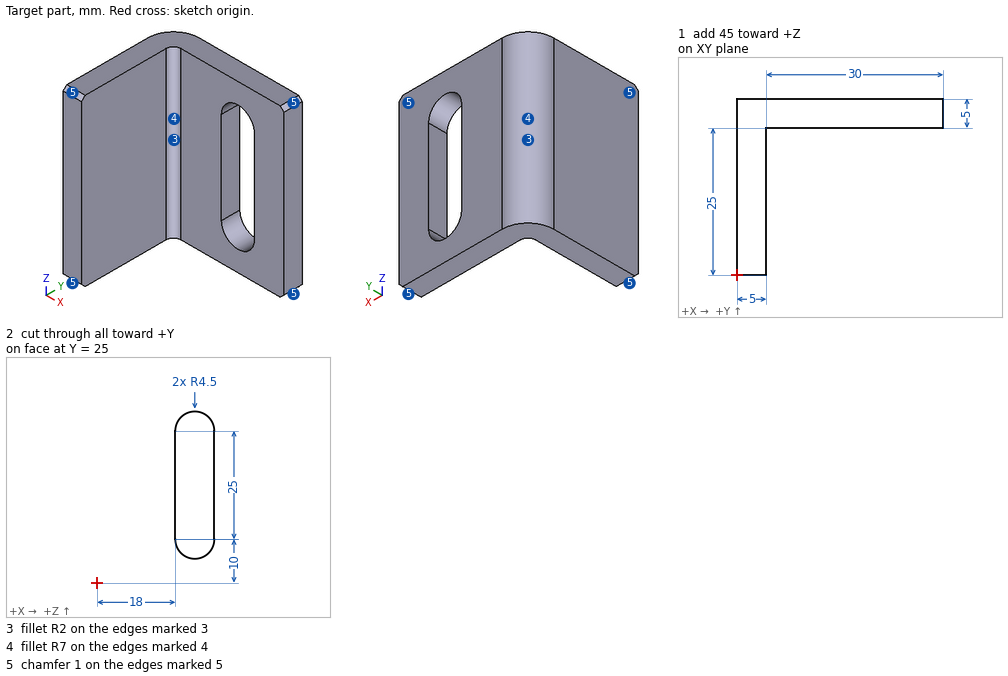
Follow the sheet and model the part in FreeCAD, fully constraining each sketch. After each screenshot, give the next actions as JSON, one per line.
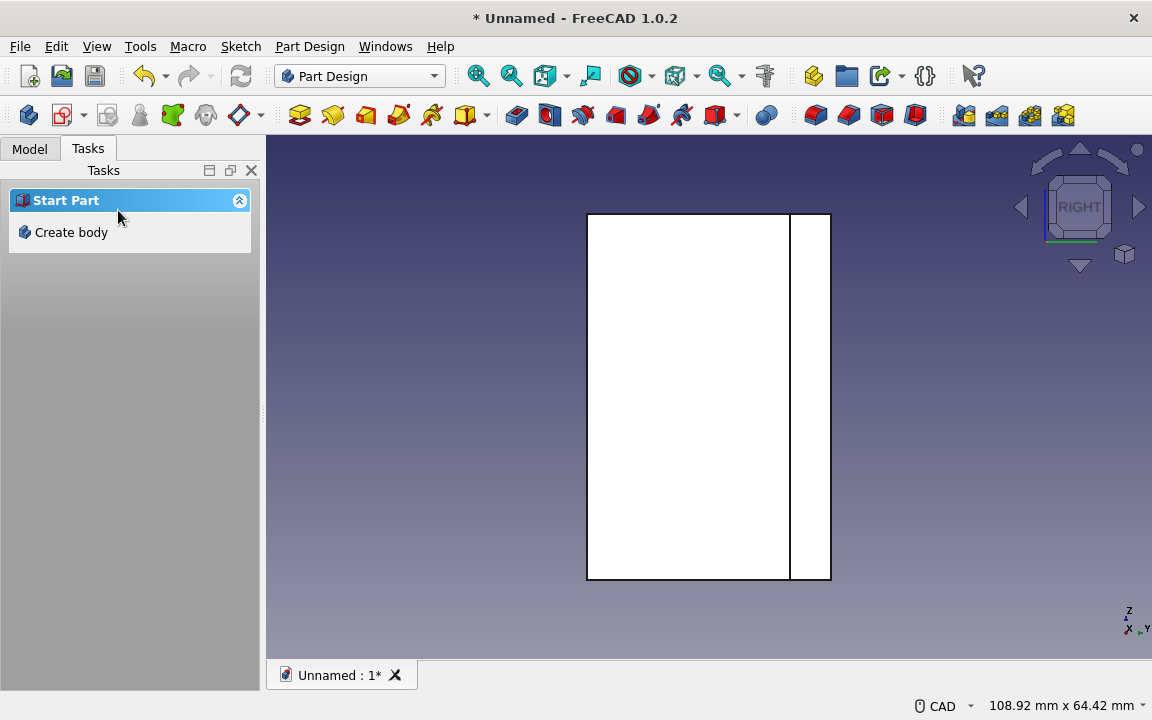
{"action": "key", "text": "5"}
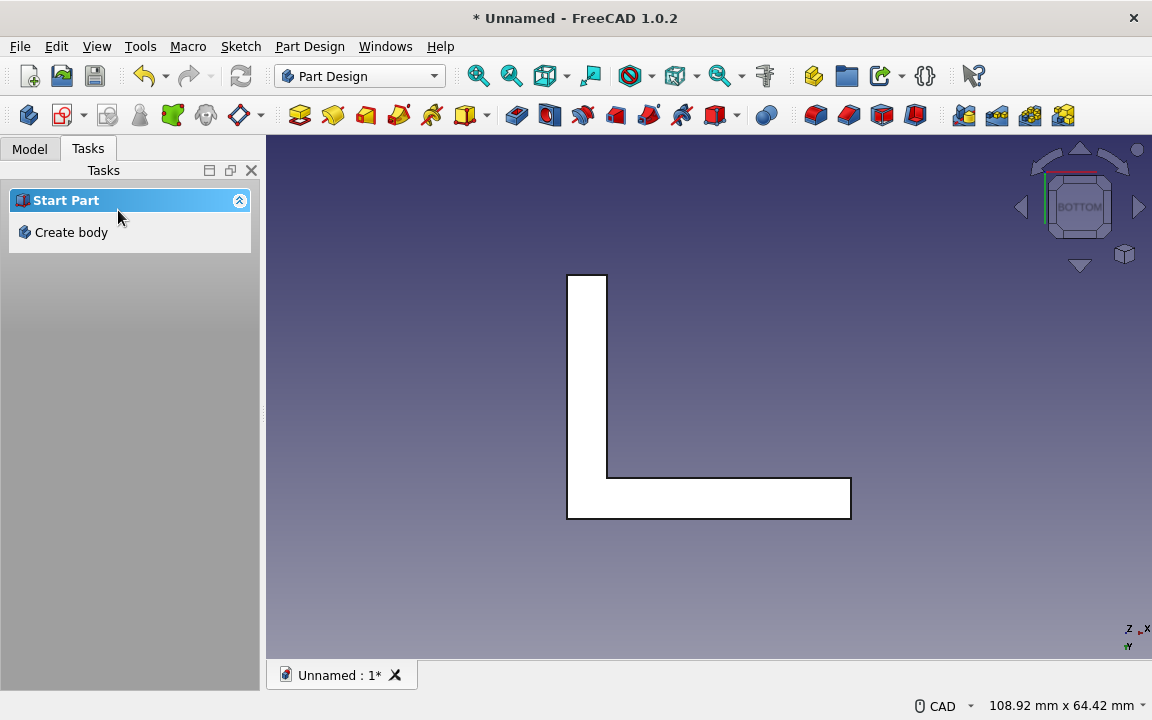
{"action": "key", "text": "4"}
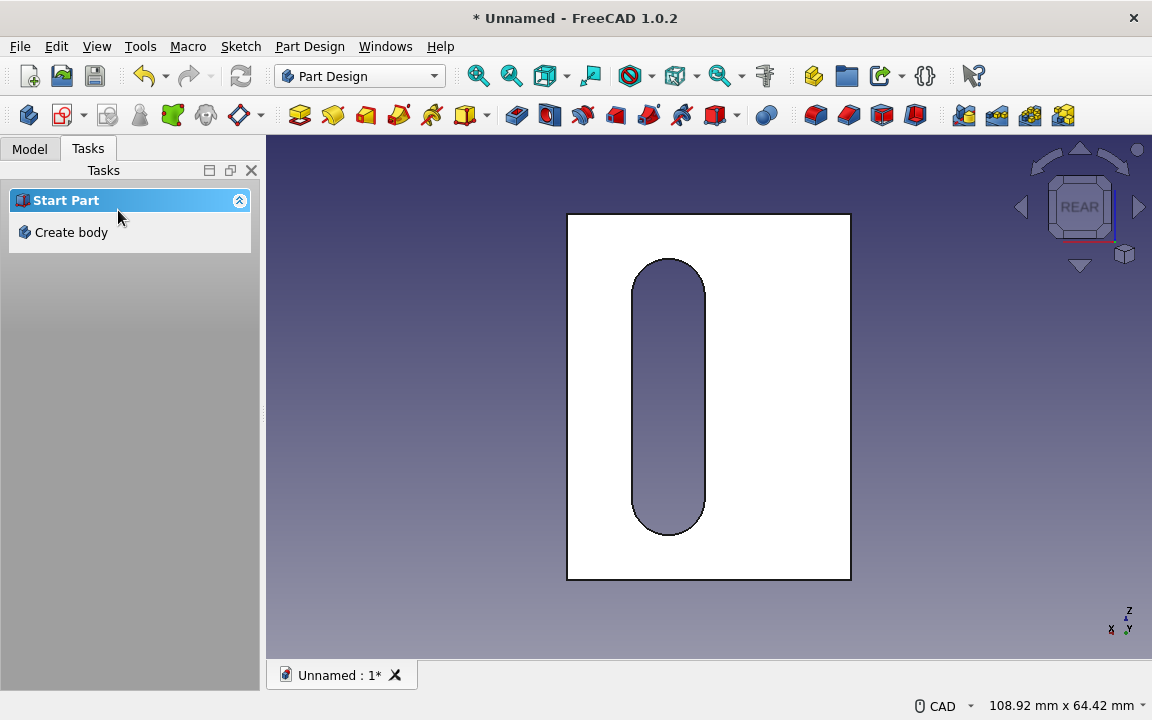
{"action": "key", "text": "6"}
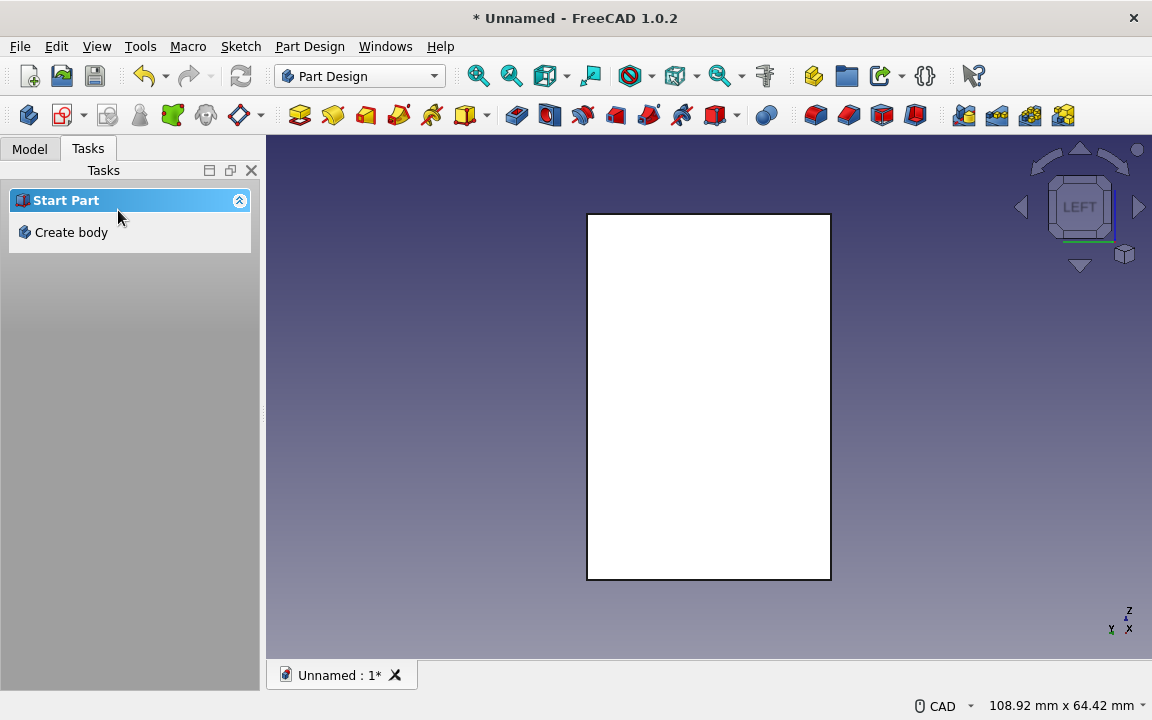
{"action": "key", "text": "v 3"}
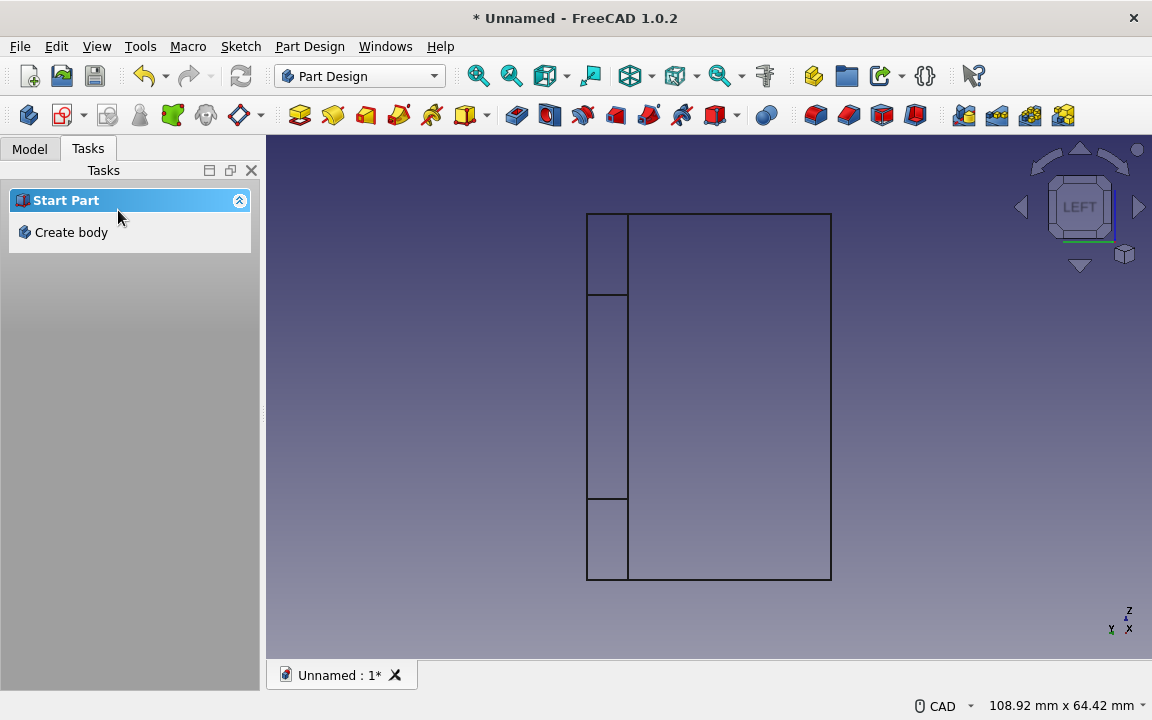
{"action": "key", "text": "0"}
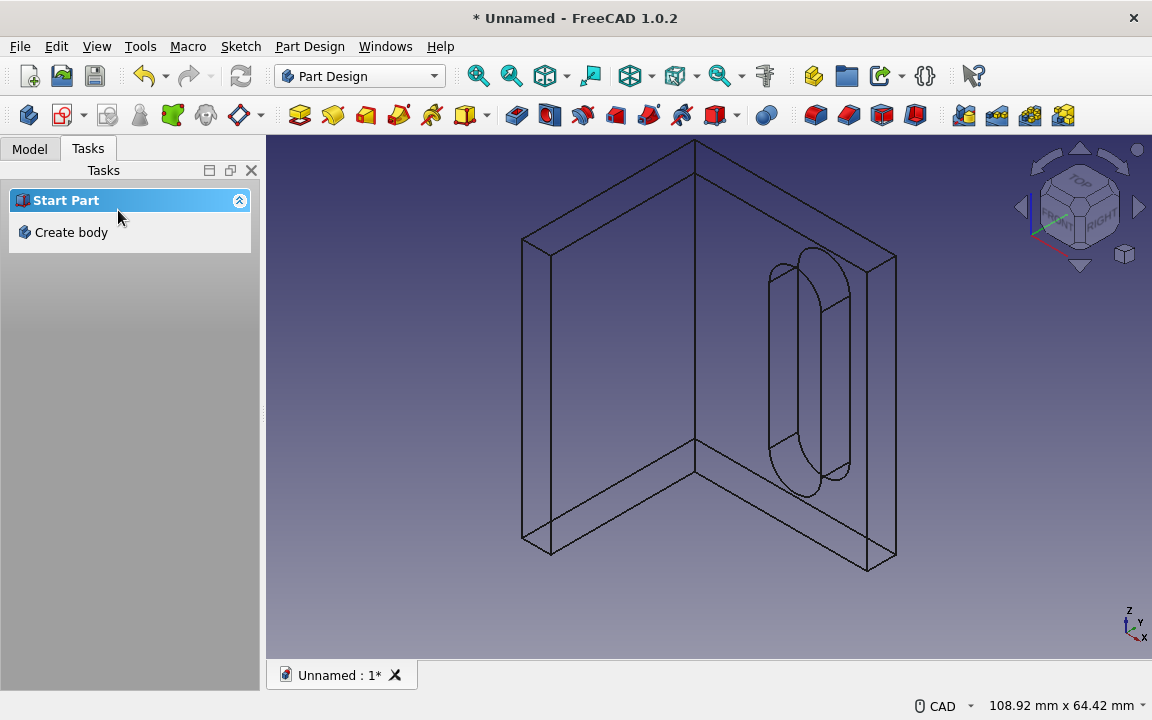
{"action": "left_click", "coordinate": [695, 321]}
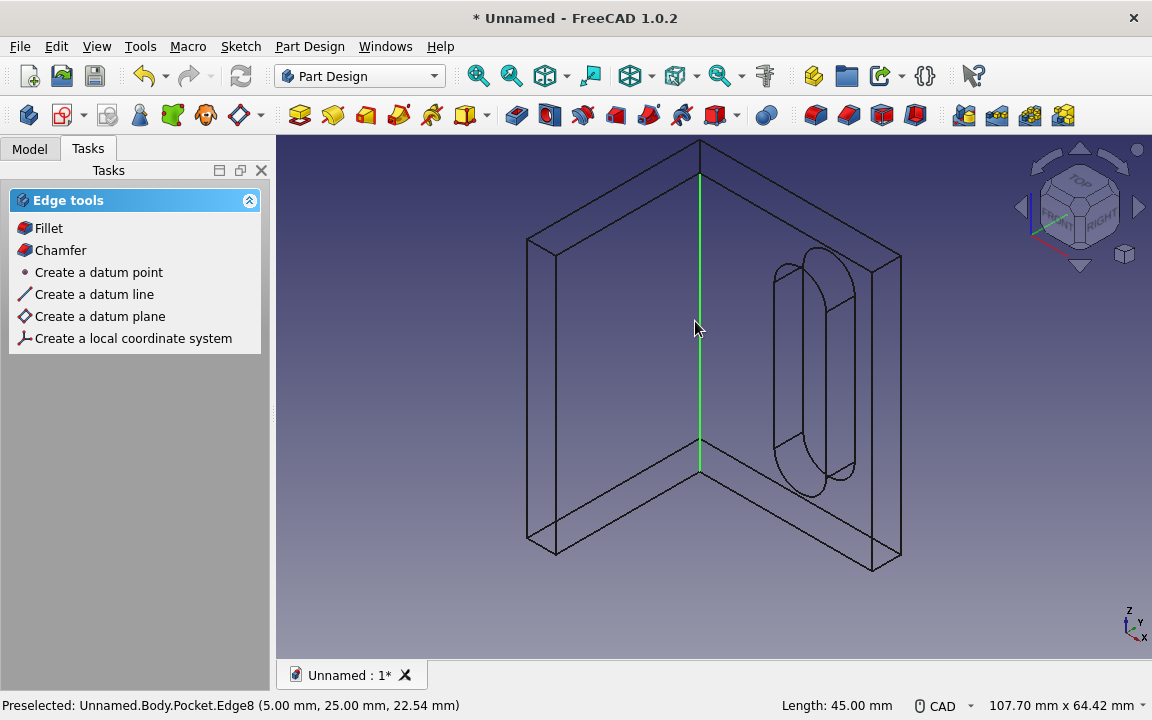
{"action": "key", "text": "v 1"}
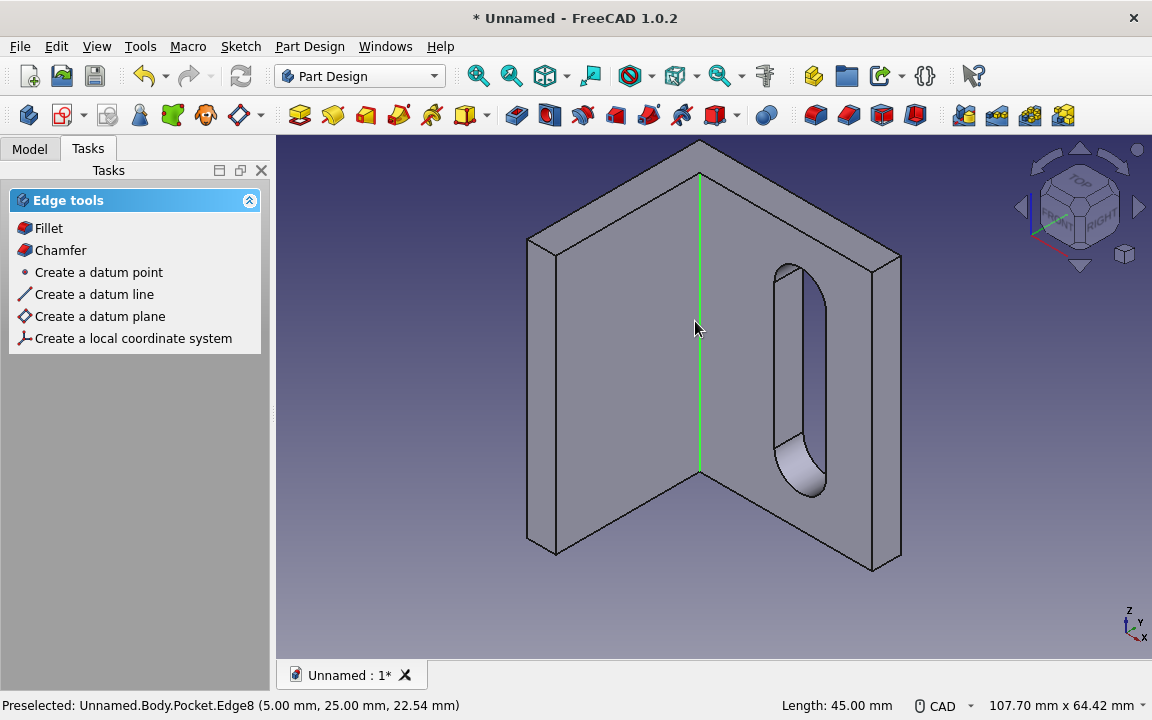
{"action": "left_click", "coordinate": [816, 116]}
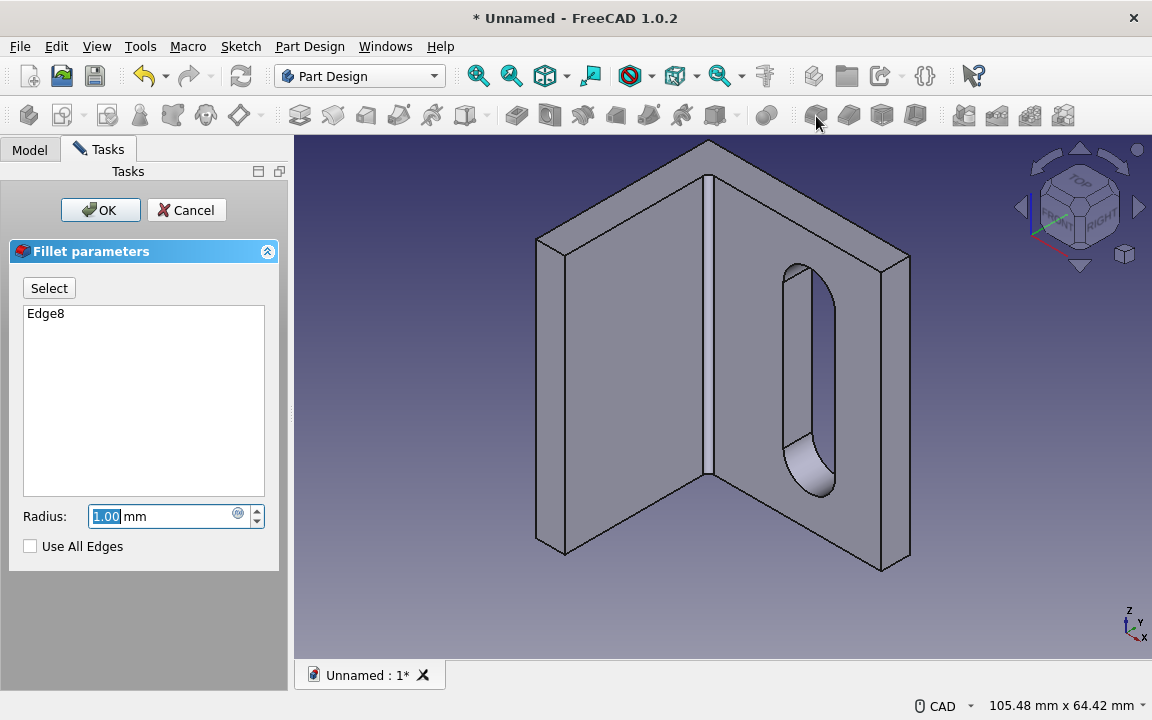
{"action": "type", "text": "2"}
{"action": "key", "text": "Tab"}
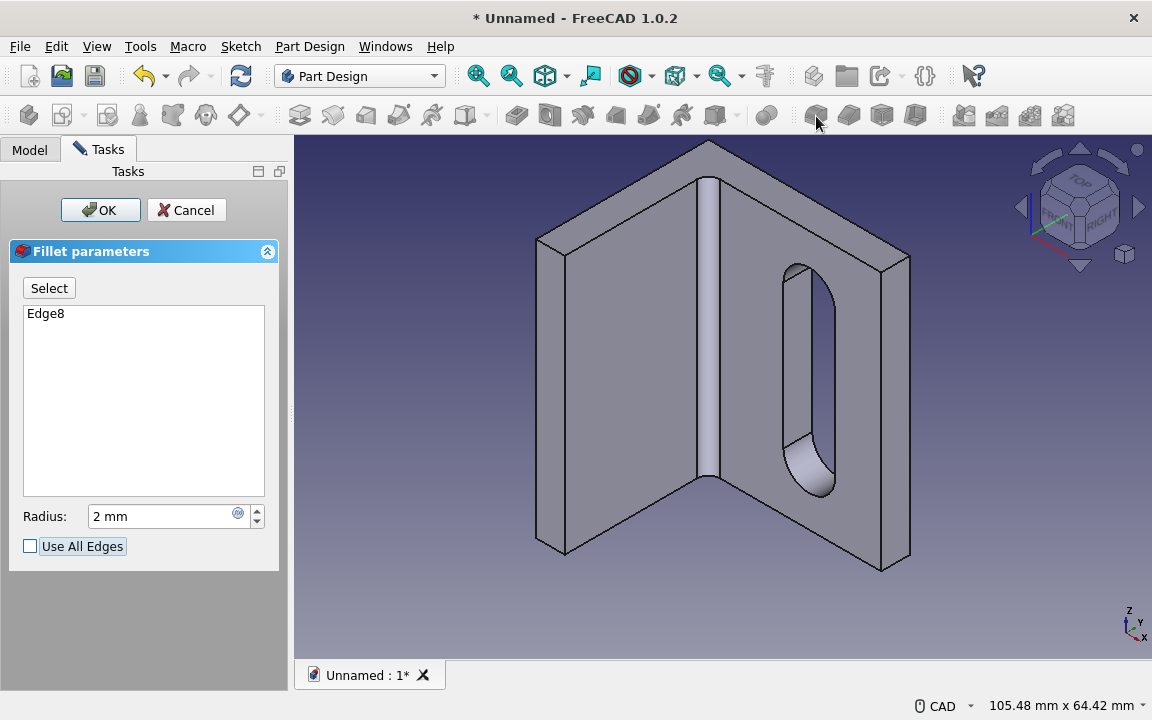
{"action": "left_click", "coordinate": [101, 210]}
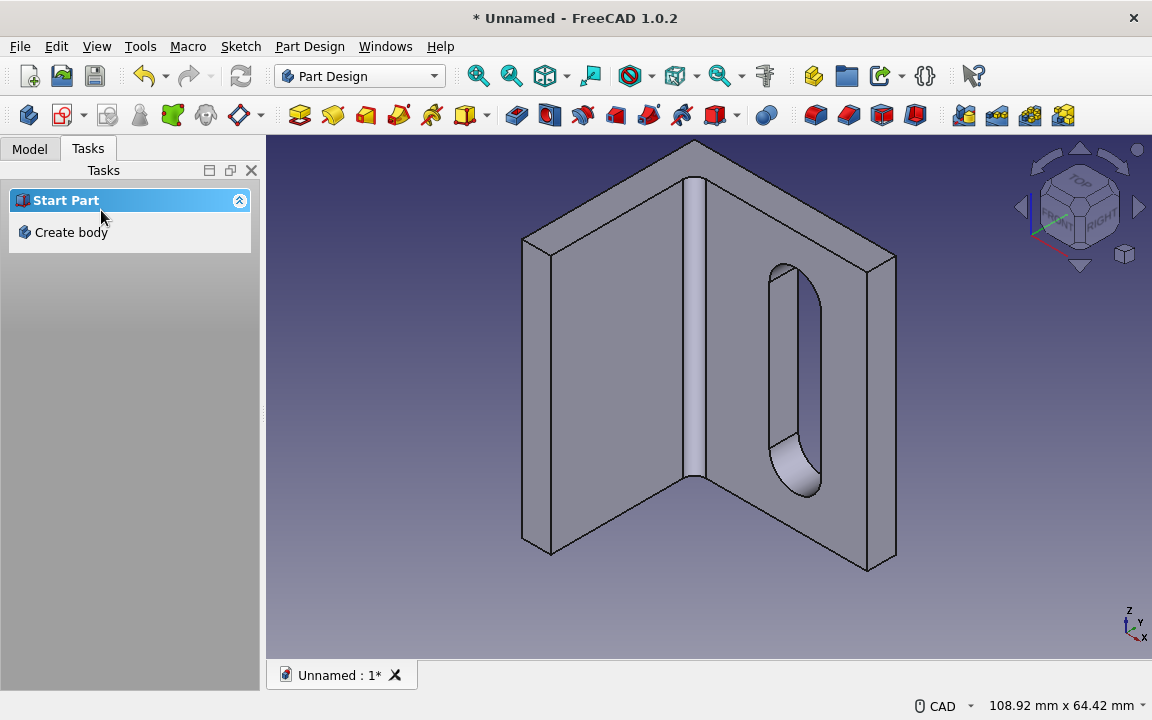
{"action": "key", "text": "2"}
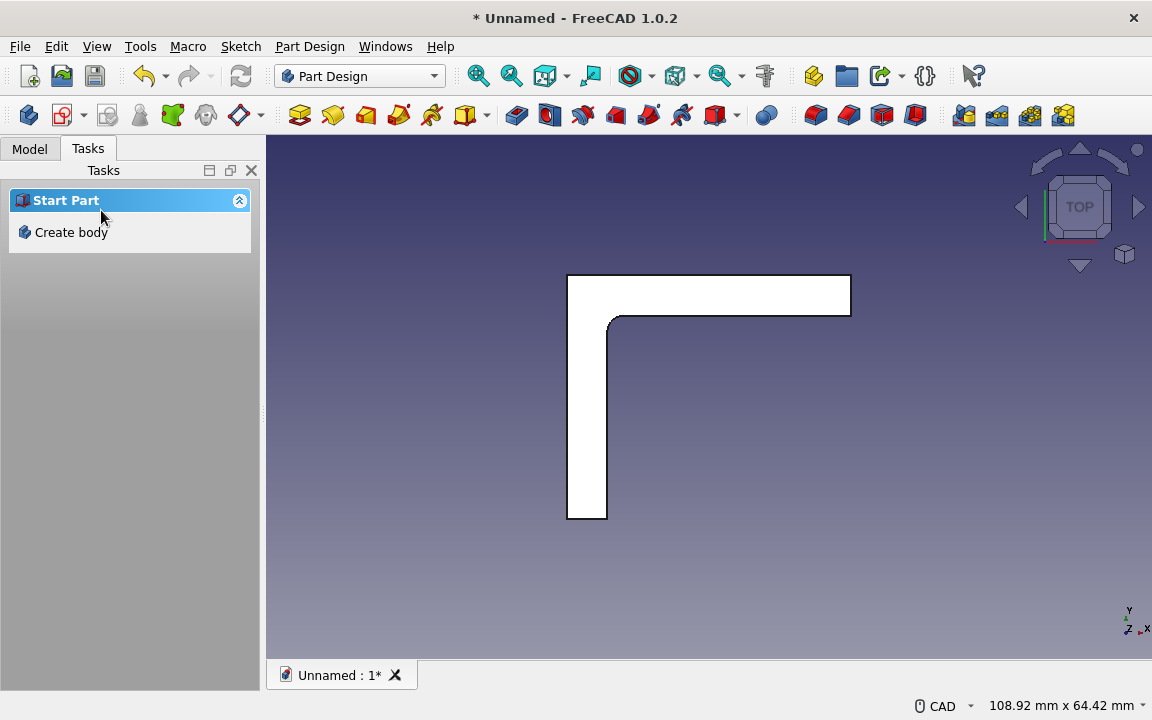
{"action": "key", "text": "0"}